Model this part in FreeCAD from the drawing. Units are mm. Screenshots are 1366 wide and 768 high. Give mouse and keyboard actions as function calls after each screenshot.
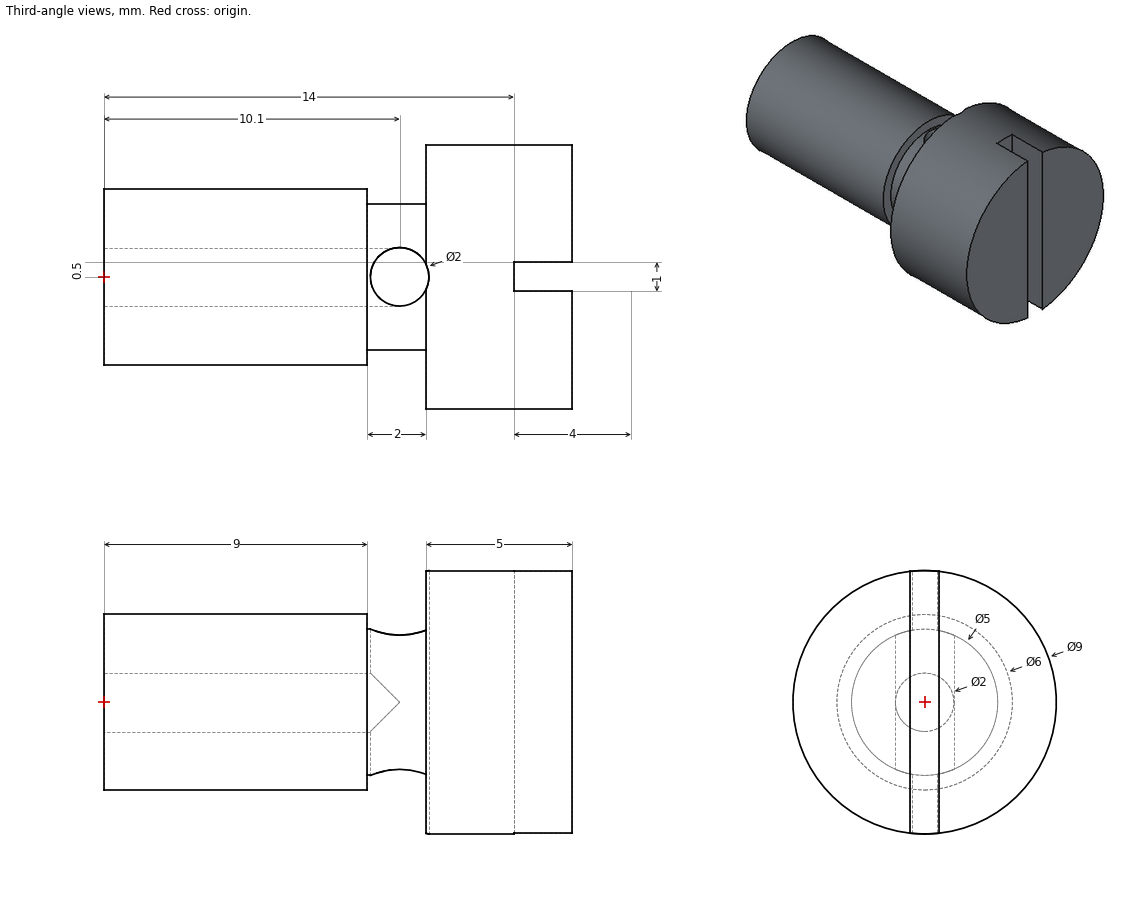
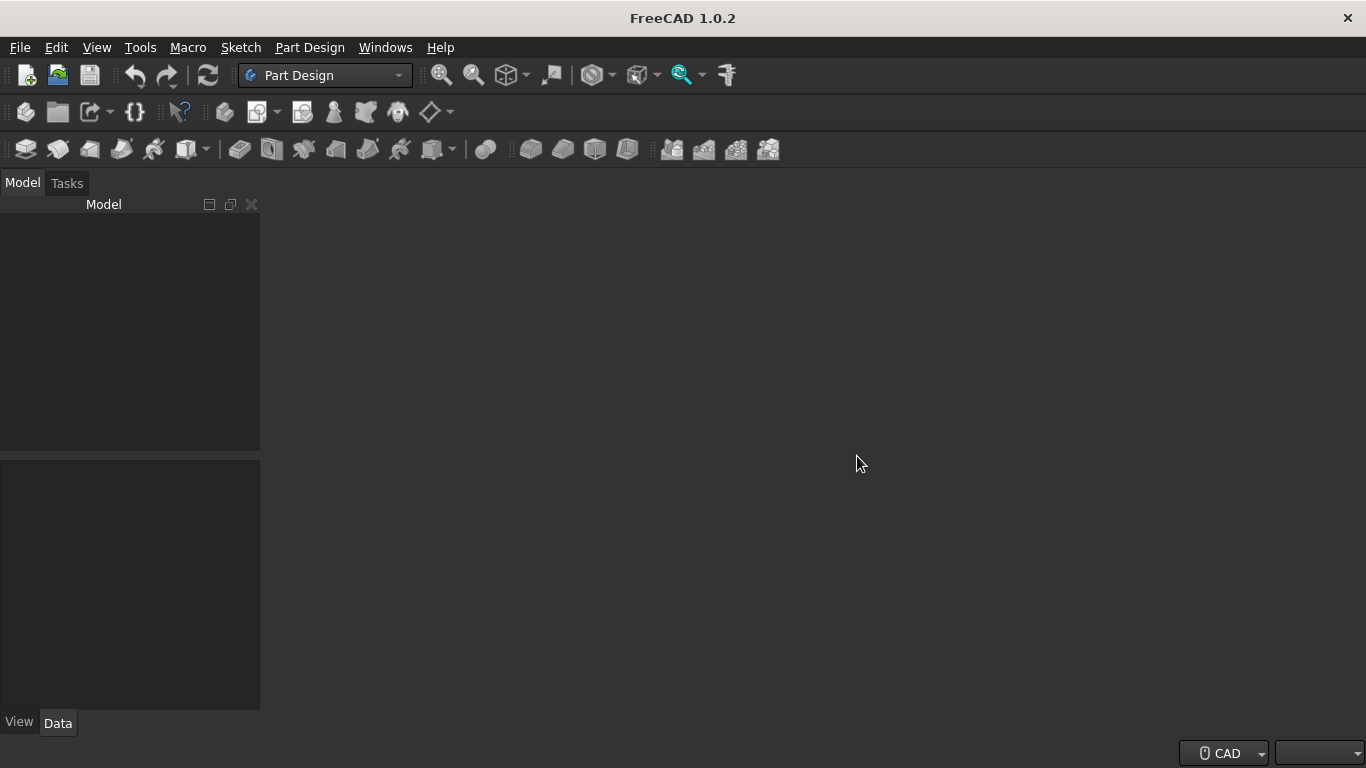
key(ctrl+n)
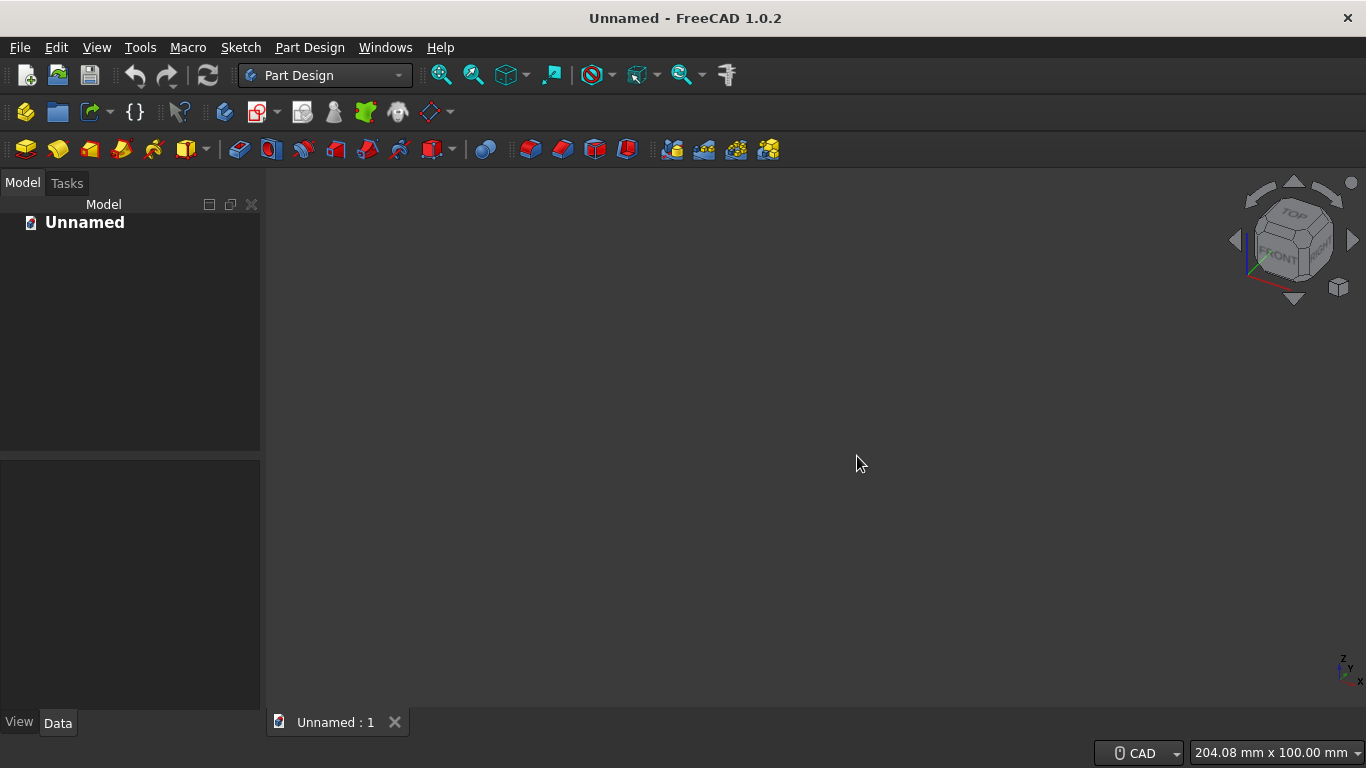
click(258, 112)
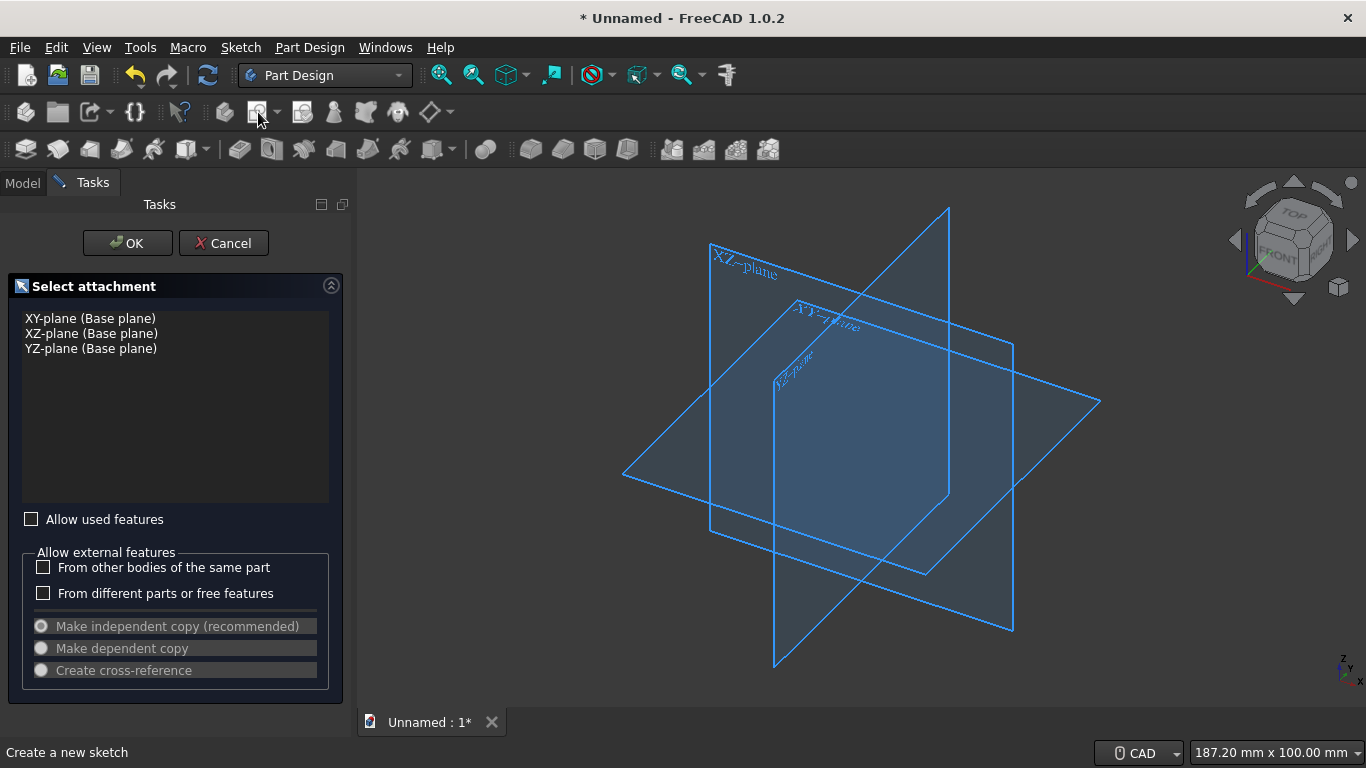
click(82, 348)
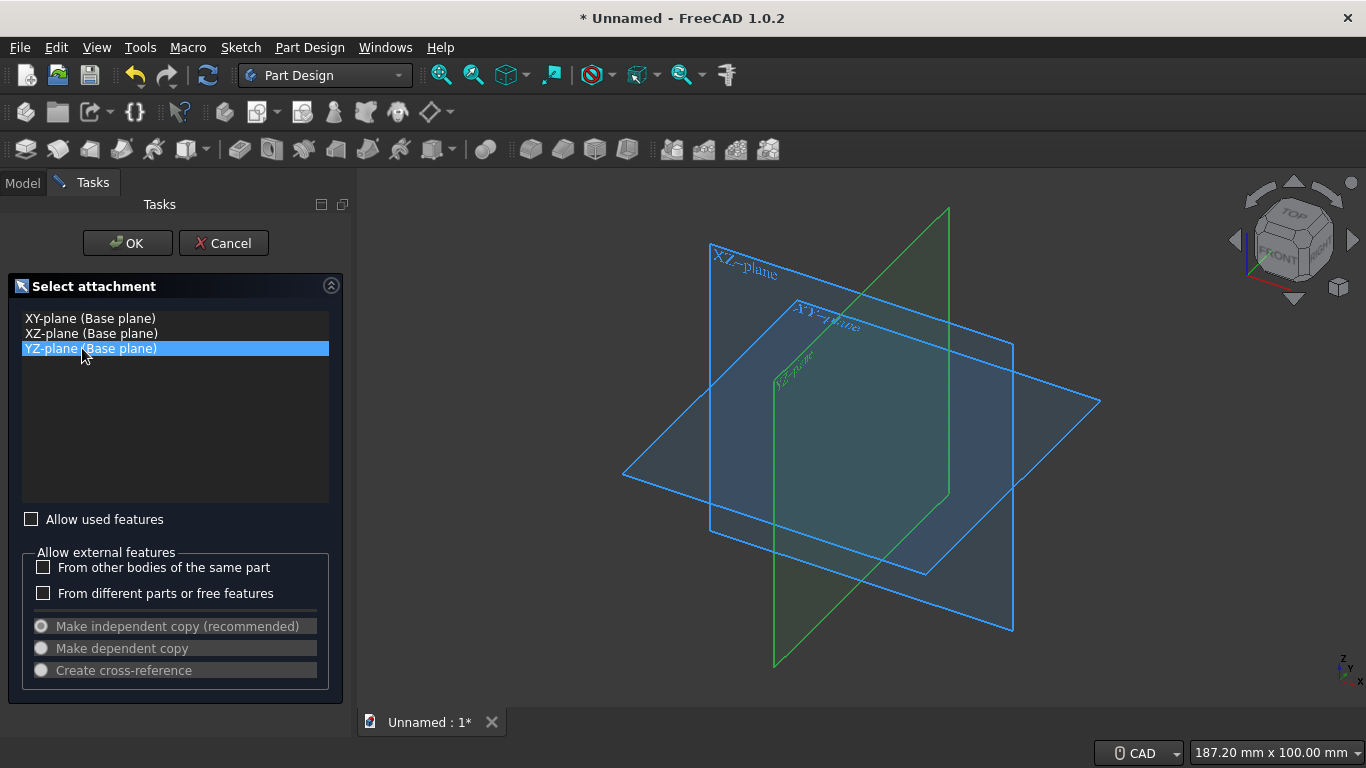
click(128, 243)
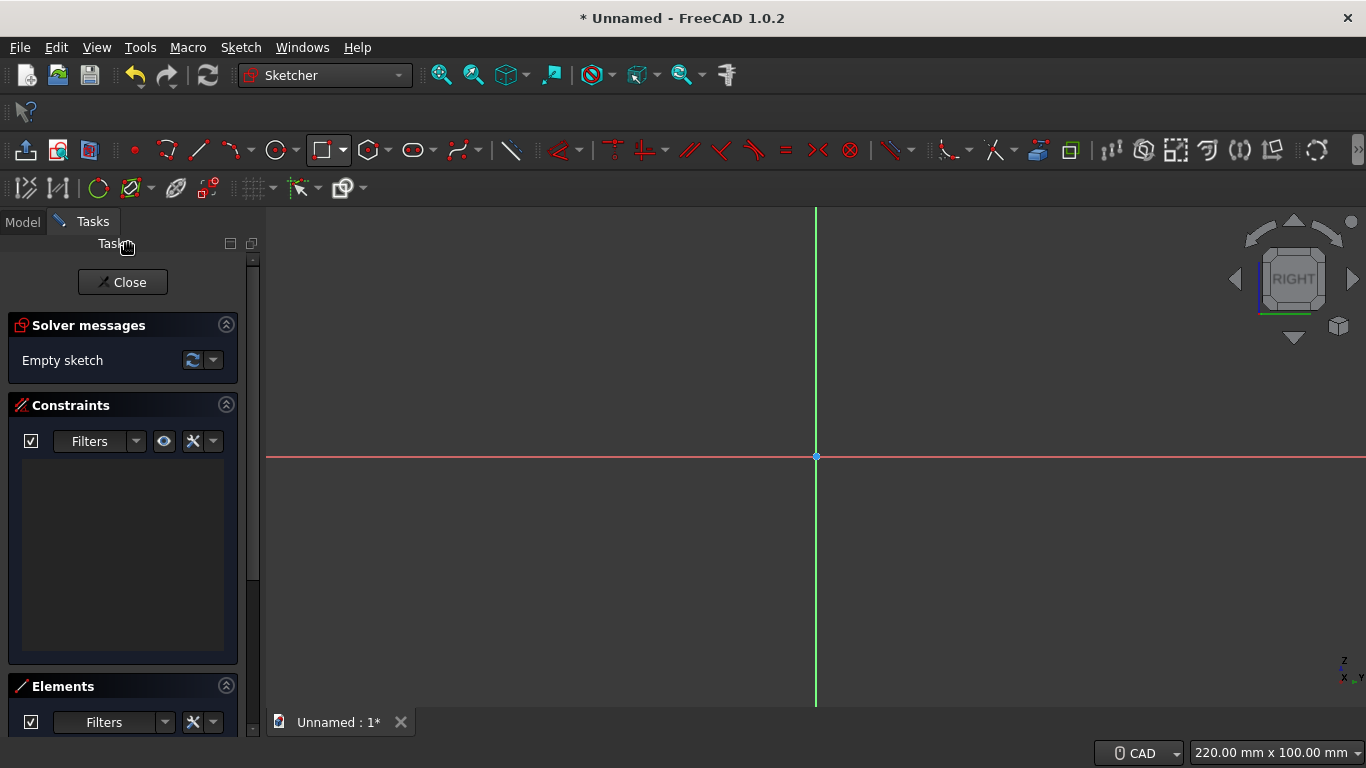
scroll(823, 457, up, 12)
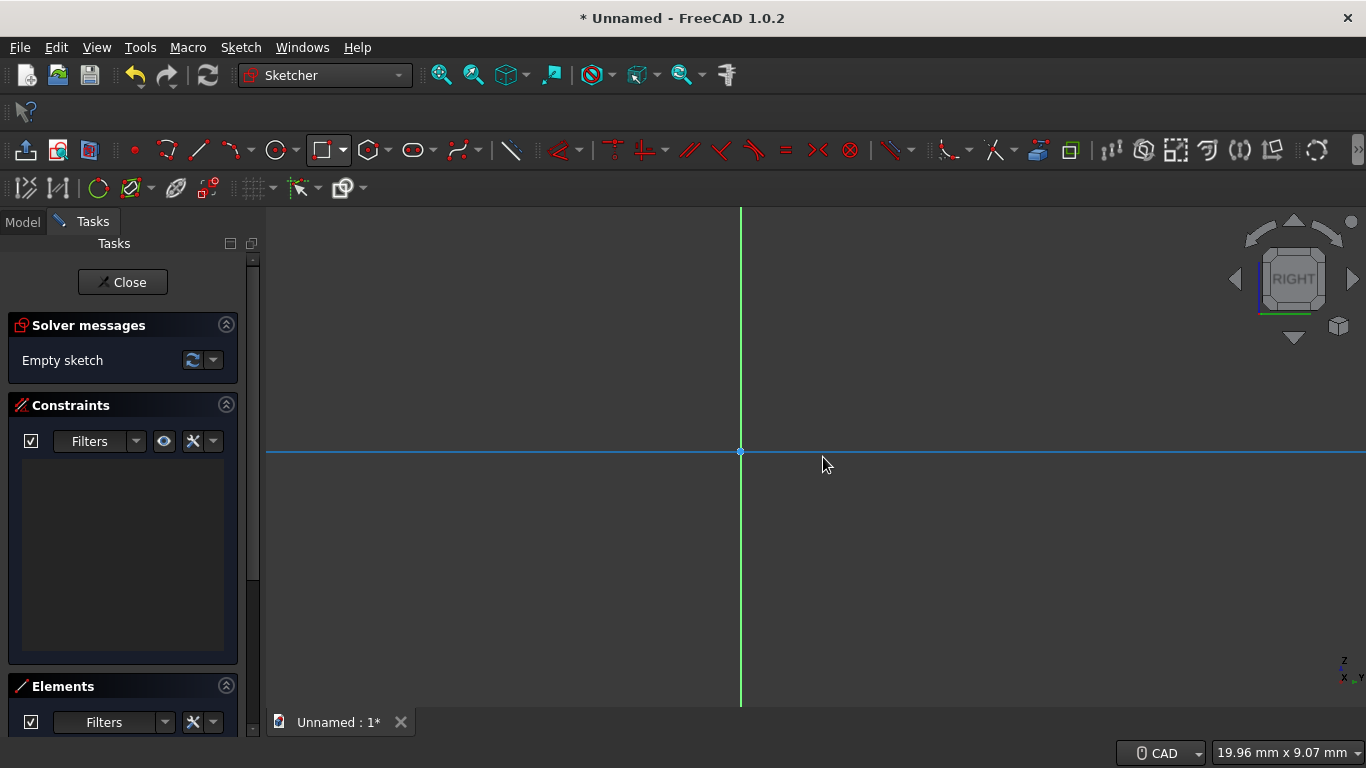
click(276, 150)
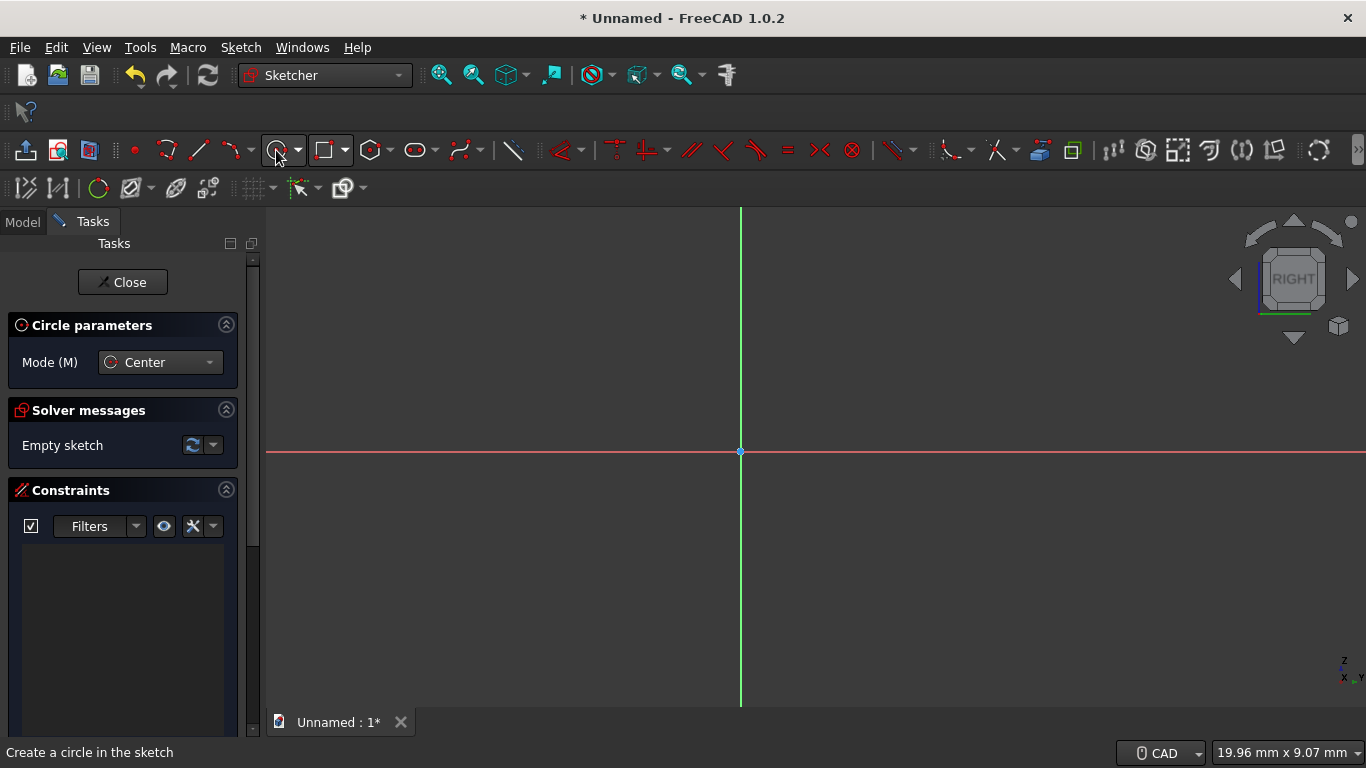
click(741, 452)
click(858, 335)
key(Escape)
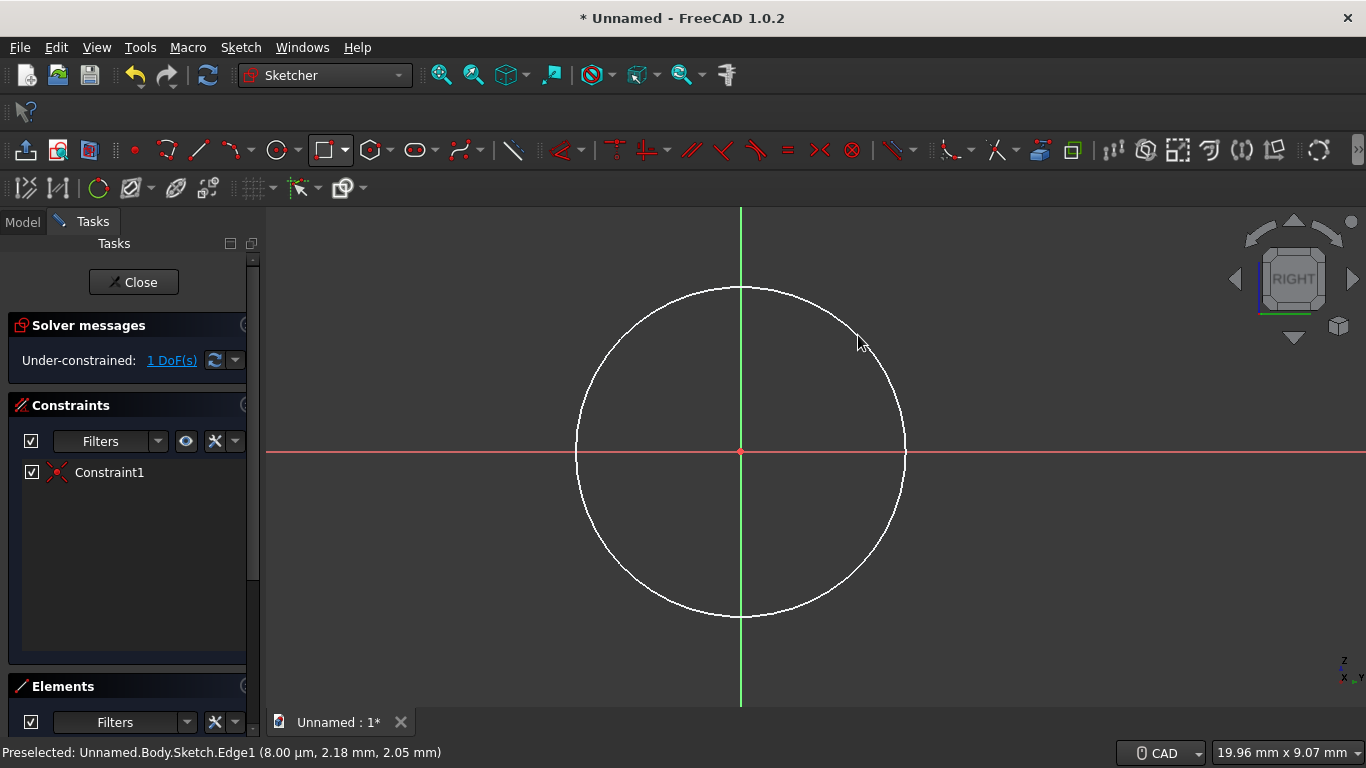
click(857, 335)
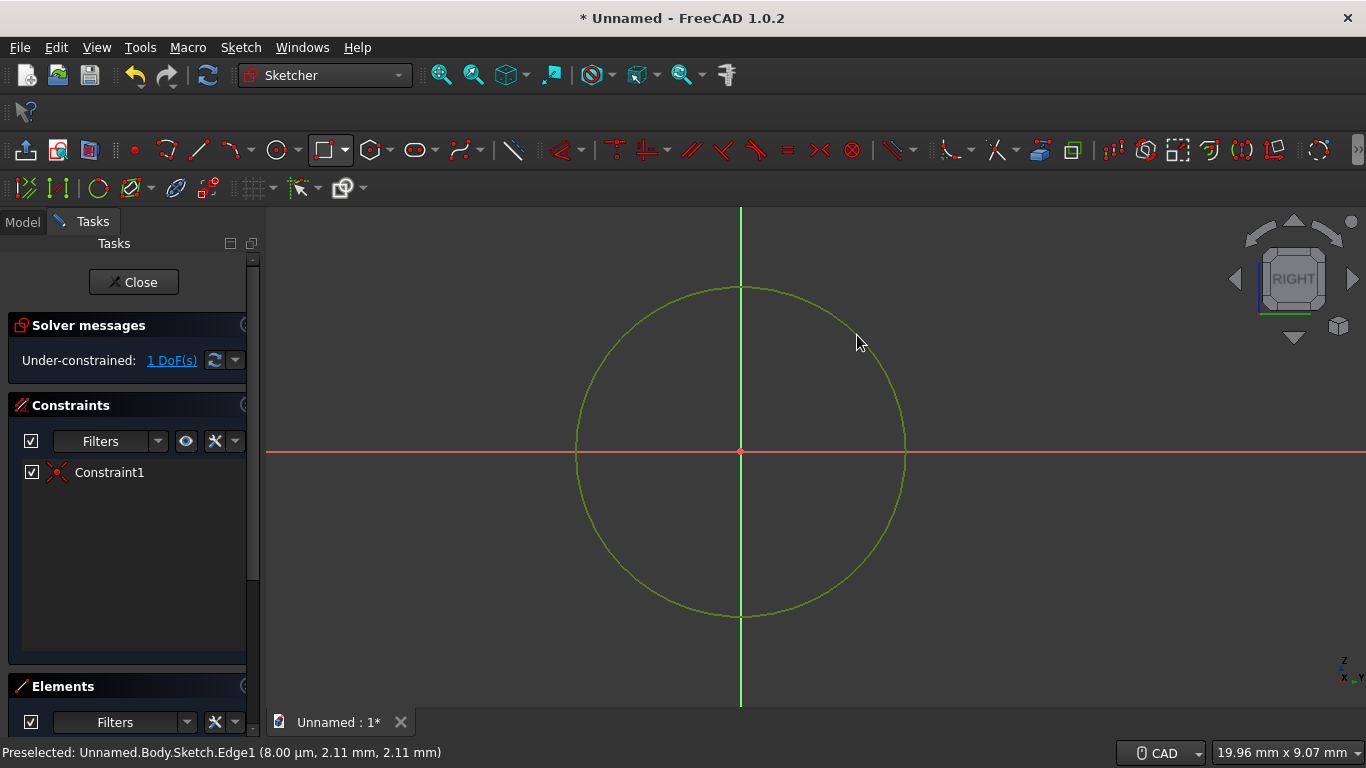
click(584, 150)